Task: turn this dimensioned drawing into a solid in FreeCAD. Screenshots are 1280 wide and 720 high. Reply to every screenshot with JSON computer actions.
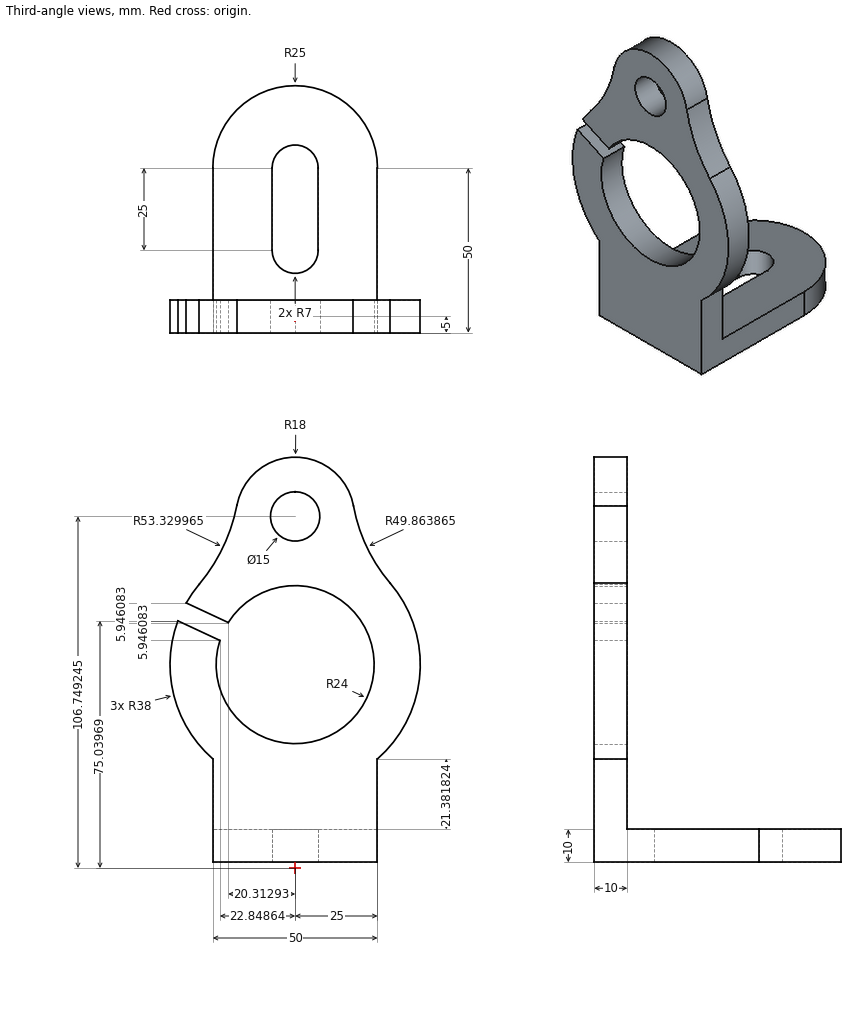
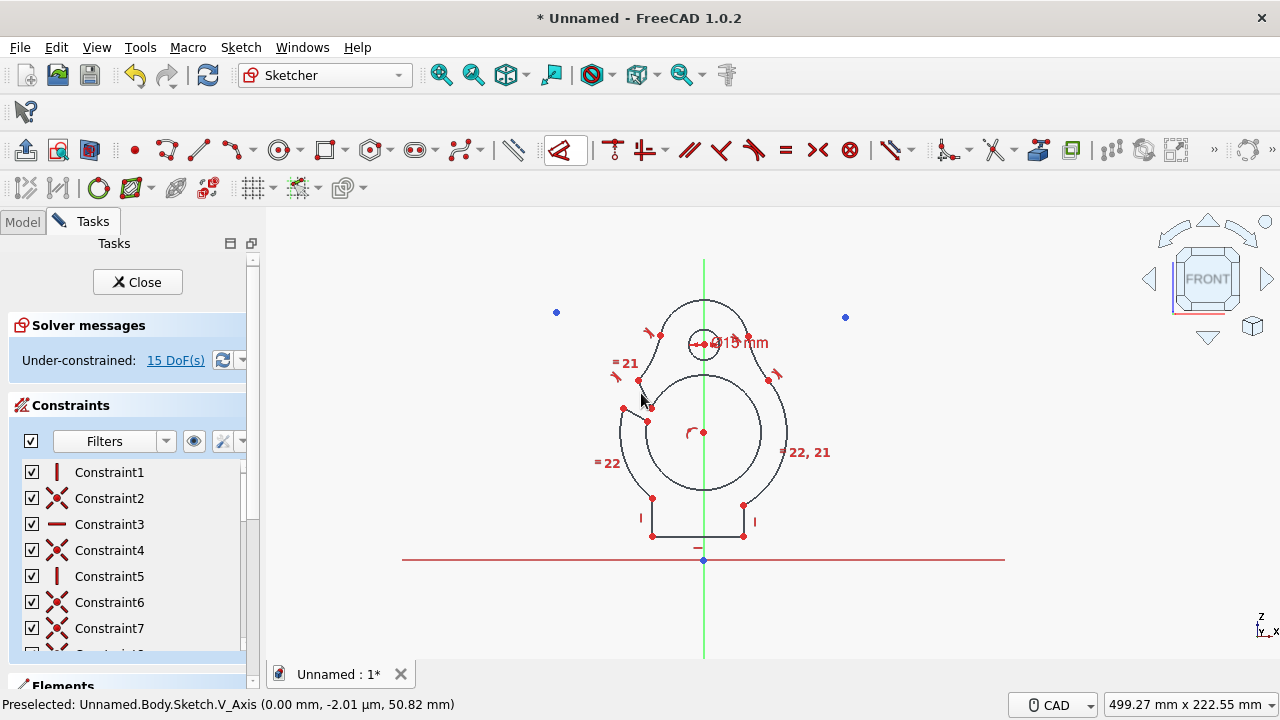
{"action": "left_click", "coordinate": [704, 345]}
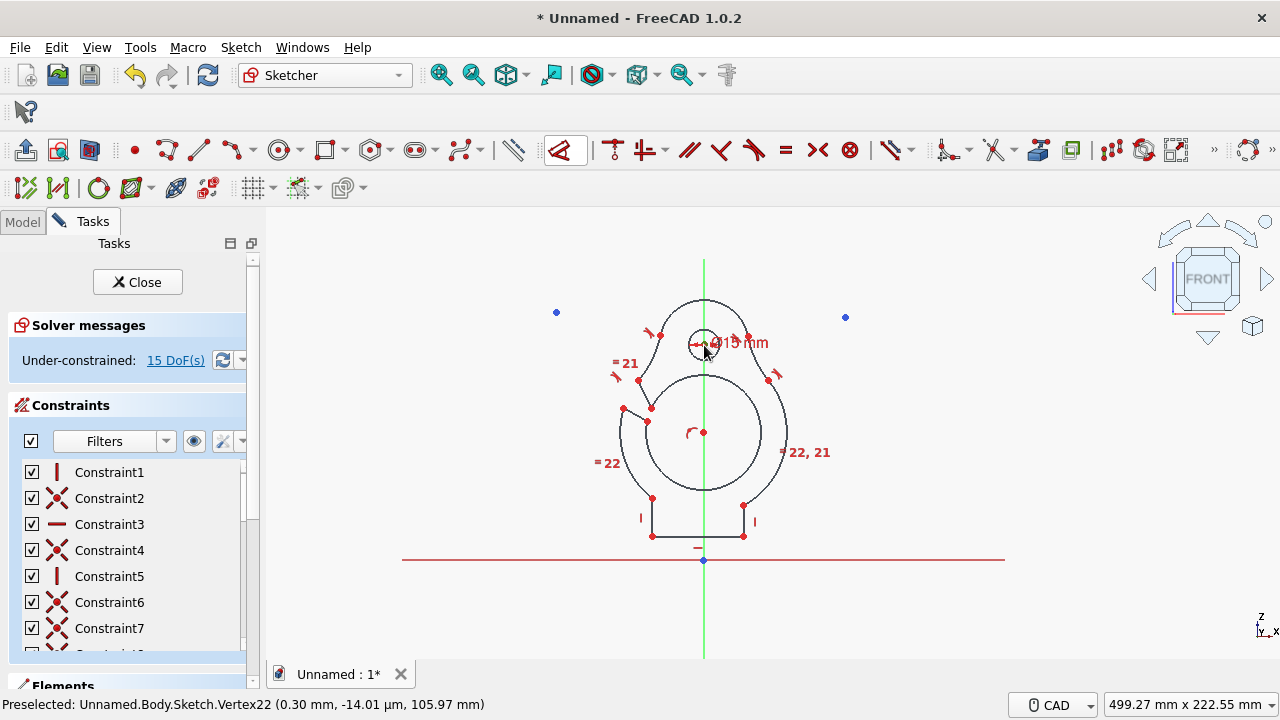
{"action": "left_click", "coordinate": [704, 603]}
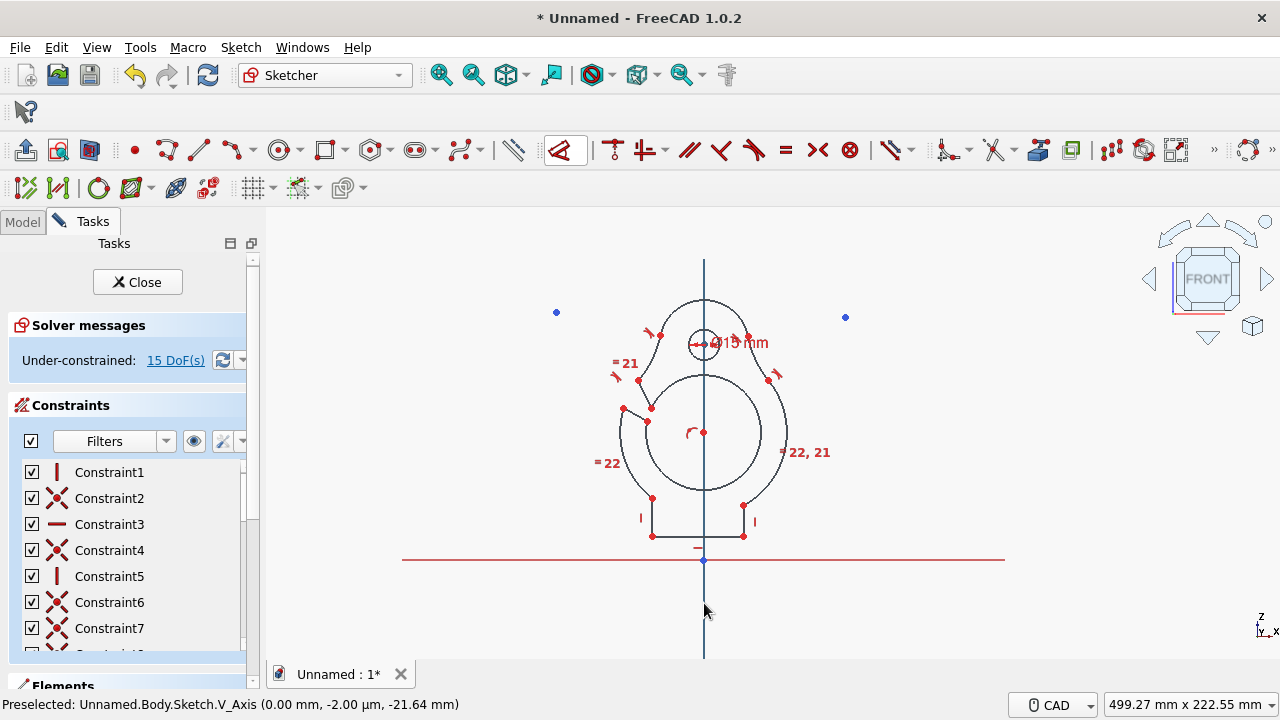
{"action": "left_click", "coordinate": [614, 150]}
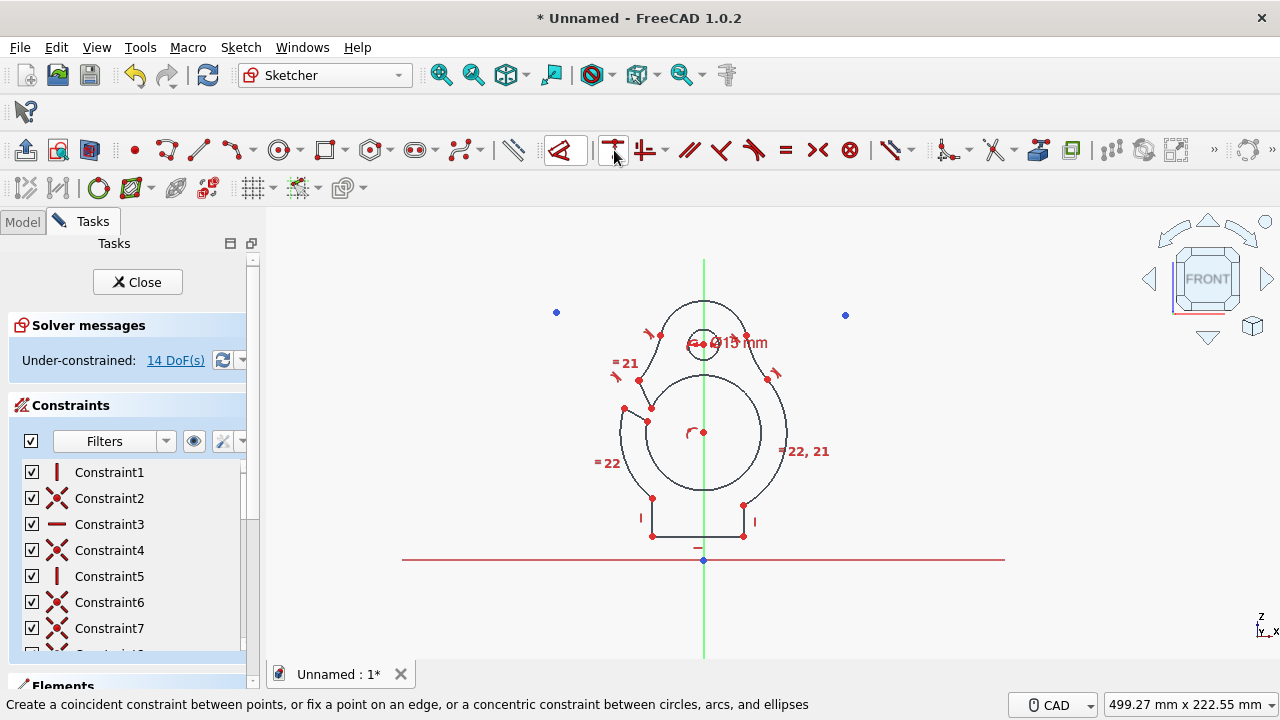
{"action": "left_click", "coordinate": [560, 150]}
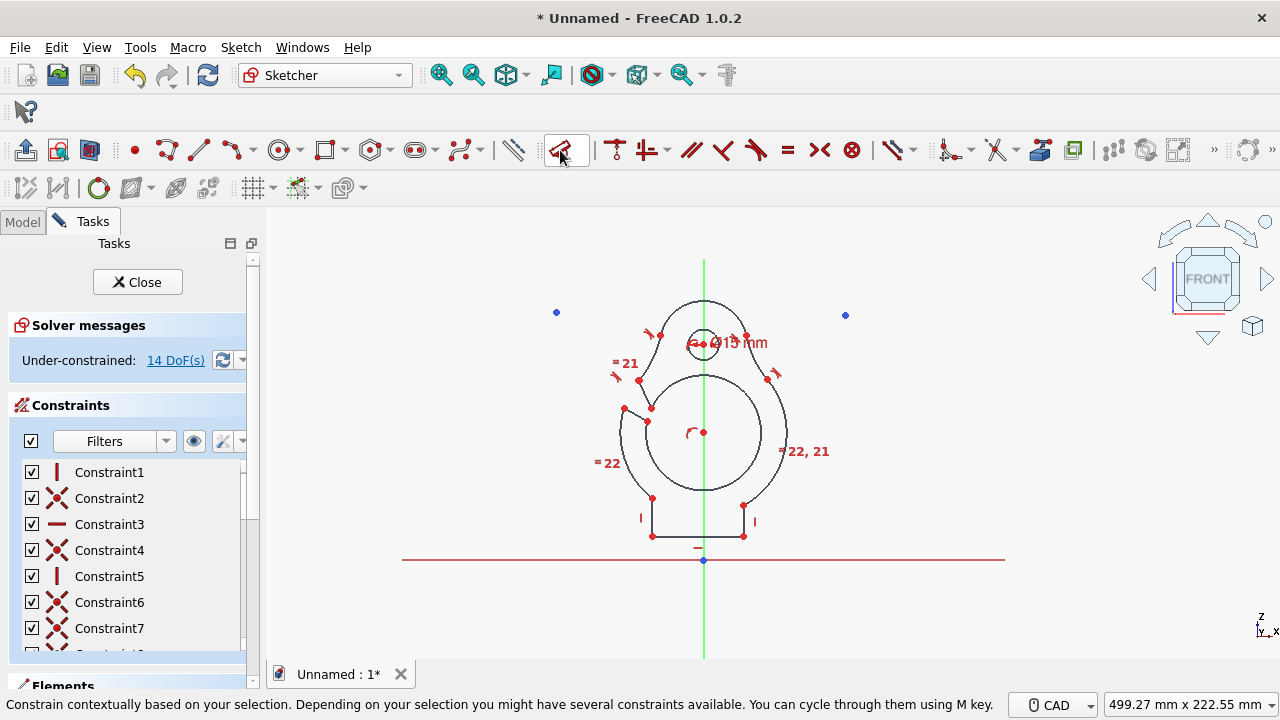
{"action": "left_click", "coordinate": [706, 490]}
{"action": "left_click", "coordinate": [762, 529]}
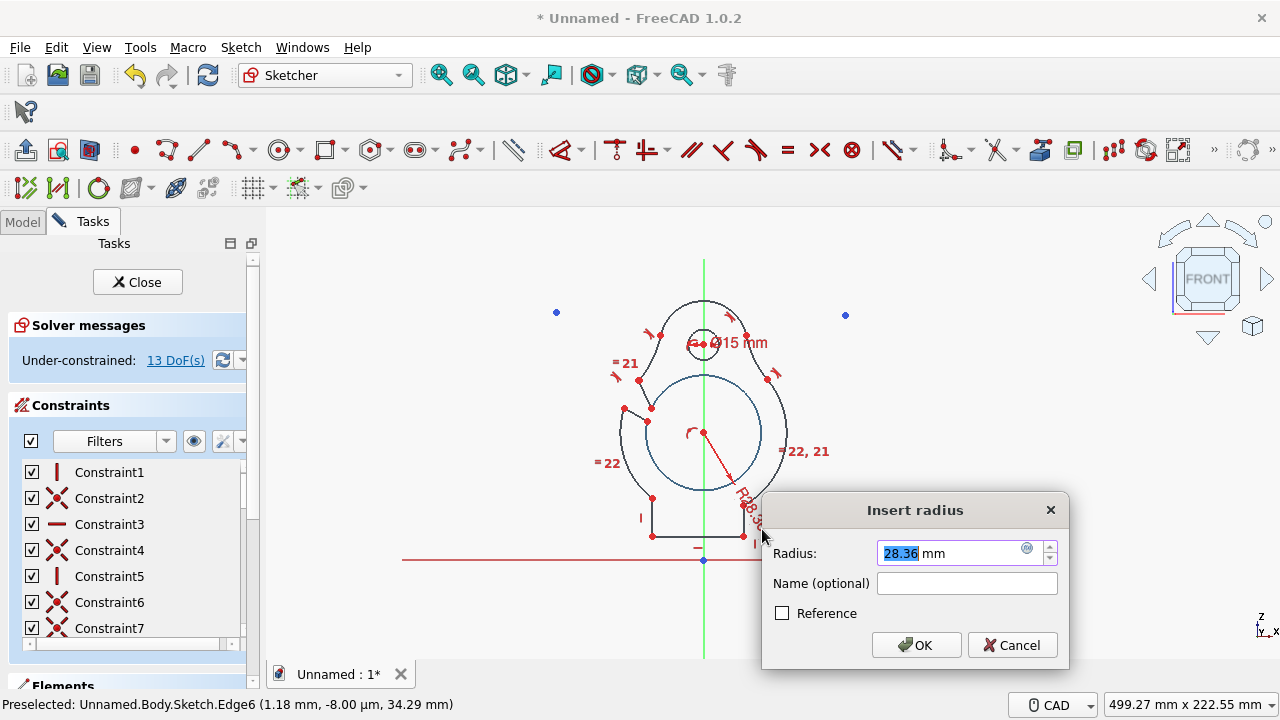
{"action": "type", "text": "24"}
{"action": "key", "text": "Return"}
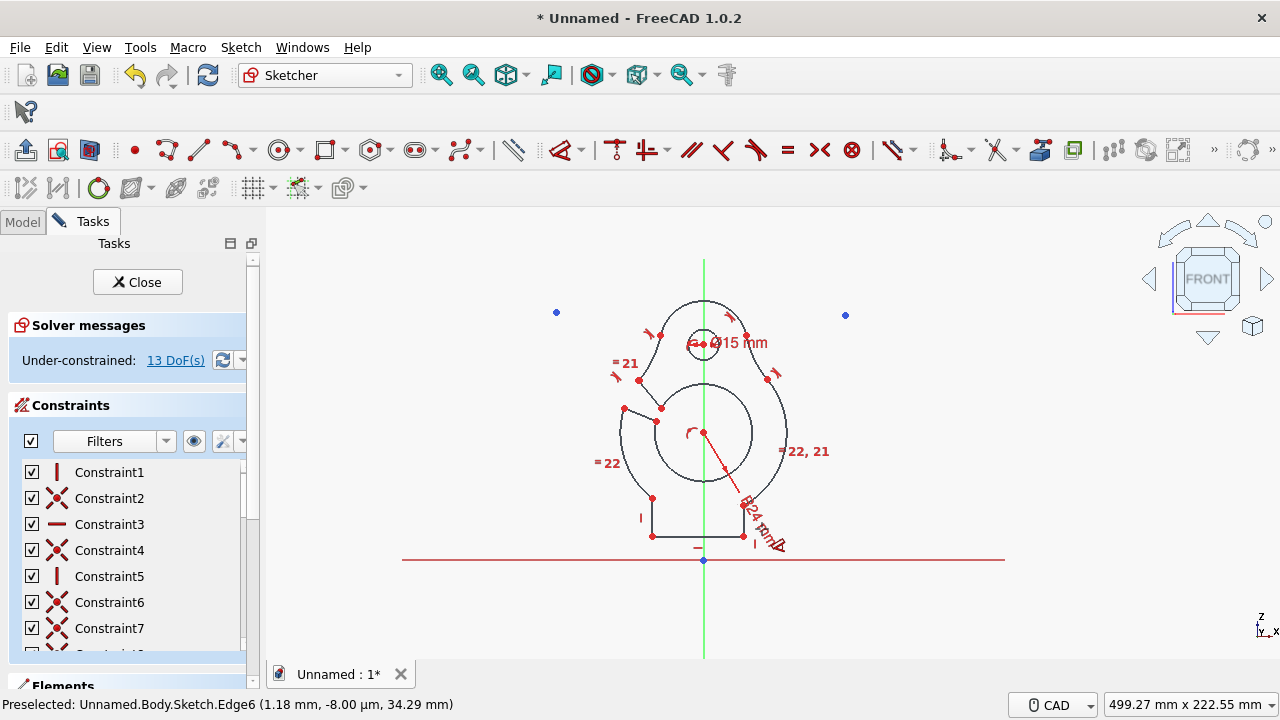
{"action": "scroll", "coordinate": [639, 381], "scroll_direction": "up", "scroll_amount": 14}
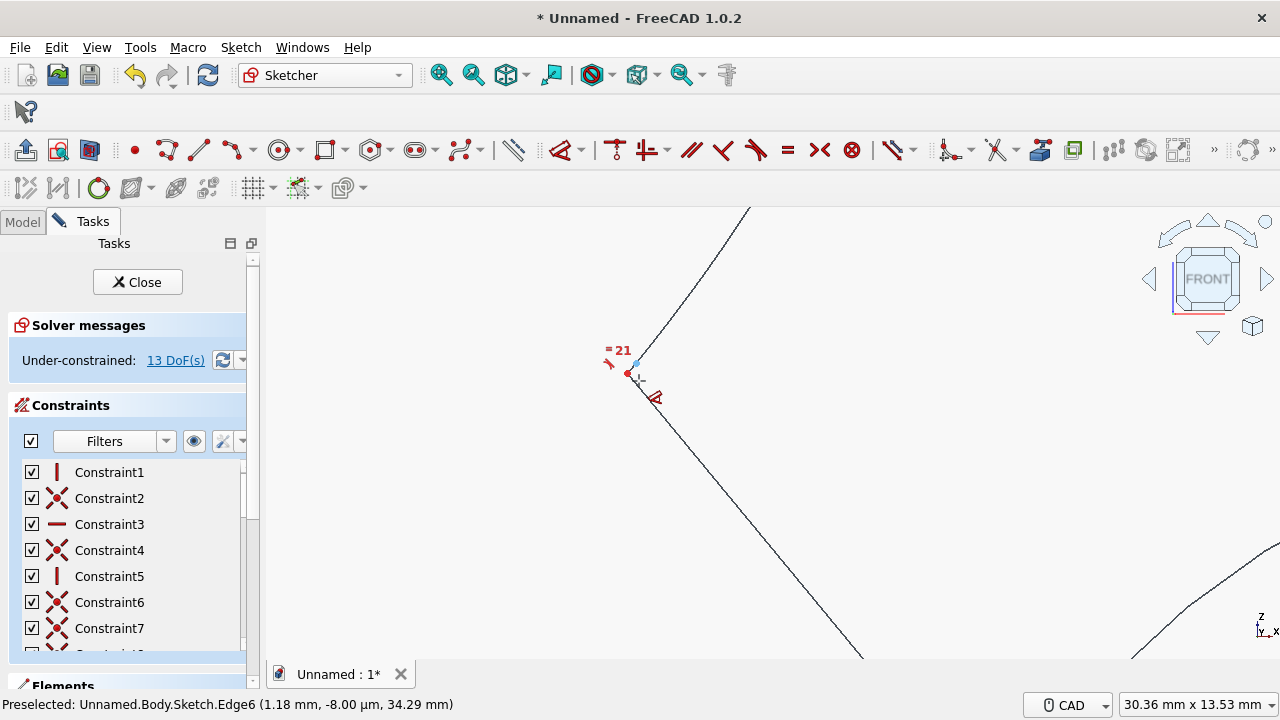
{"action": "left_click", "coordinate": [632, 368]}
{"action": "left_click", "coordinate": [607, 348]}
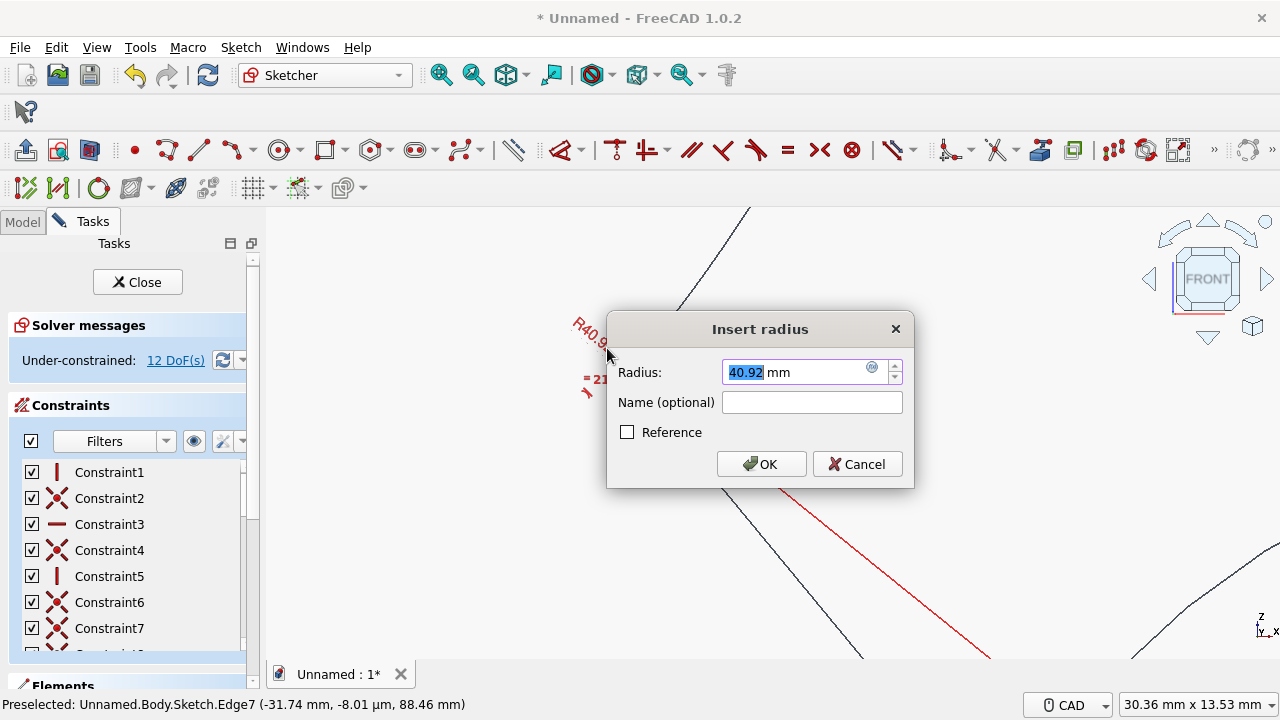
{"action": "type", "text": "38"}
{"action": "key", "text": "Return"}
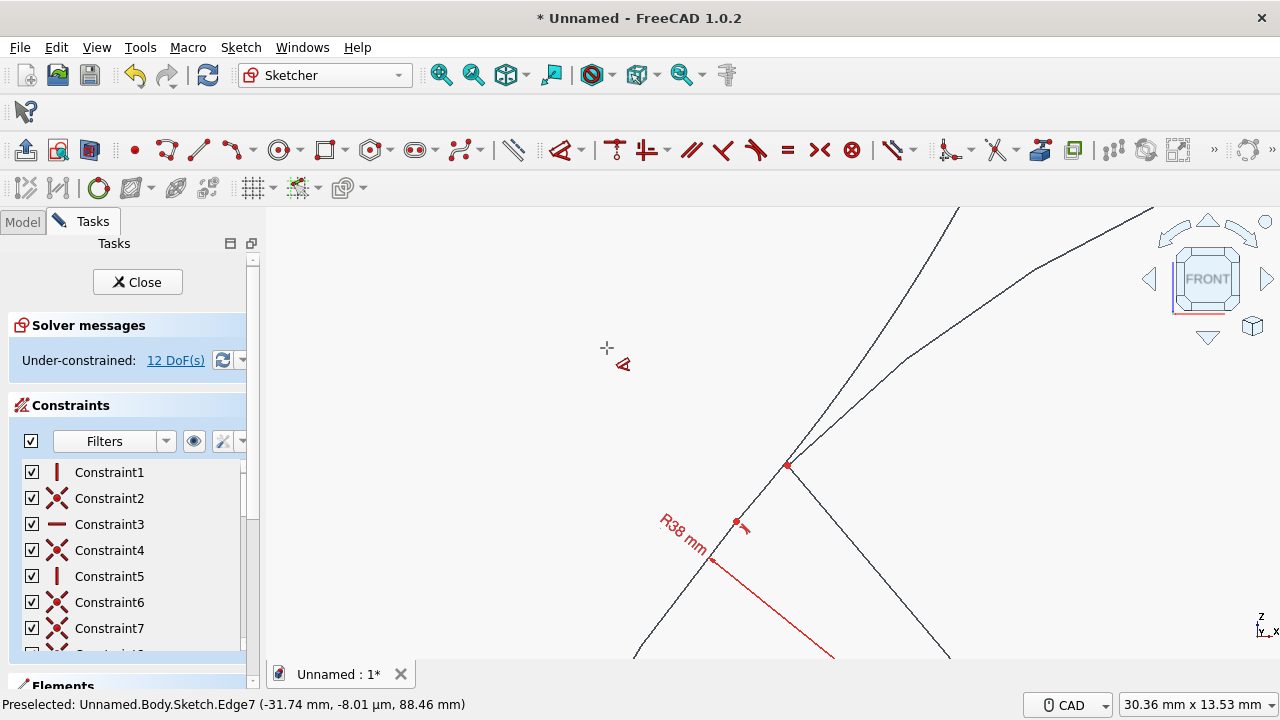
{"action": "scroll", "coordinate": [639, 381], "scroll_direction": "down", "scroll_amount": 14}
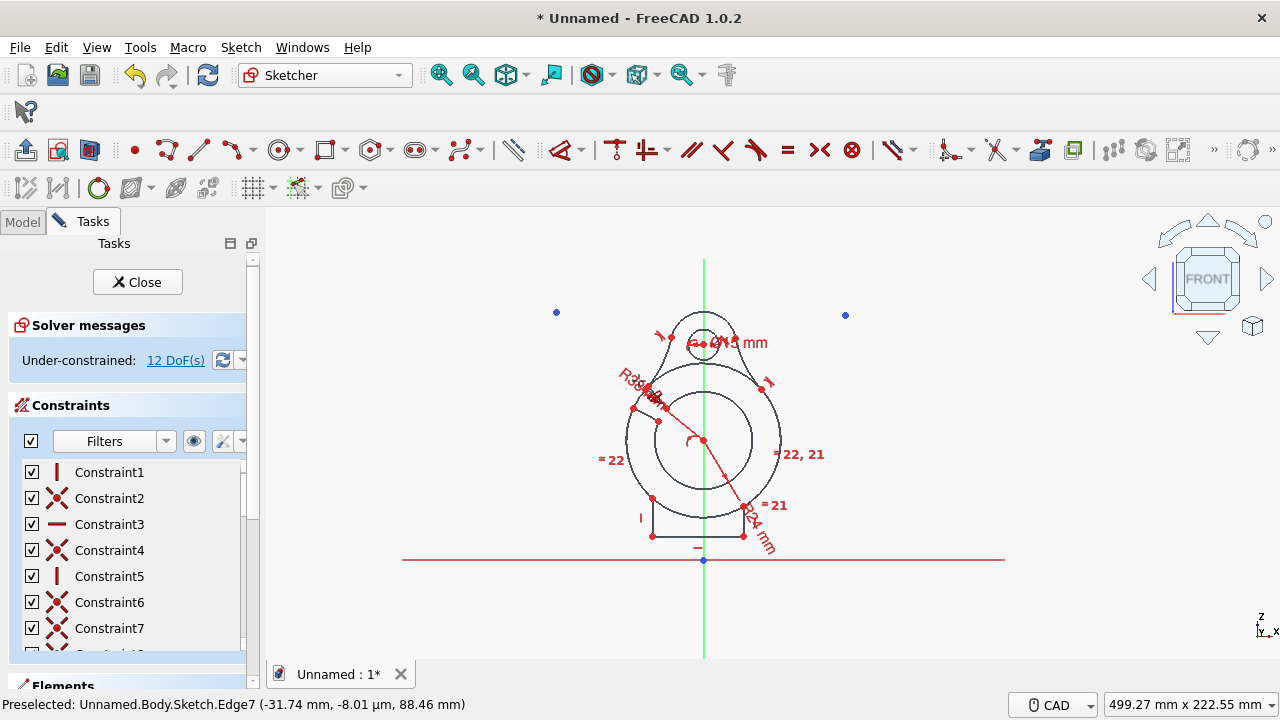
{"action": "scroll", "coordinate": [656, 376], "scroll_direction": "up", "scroll_amount": 8}